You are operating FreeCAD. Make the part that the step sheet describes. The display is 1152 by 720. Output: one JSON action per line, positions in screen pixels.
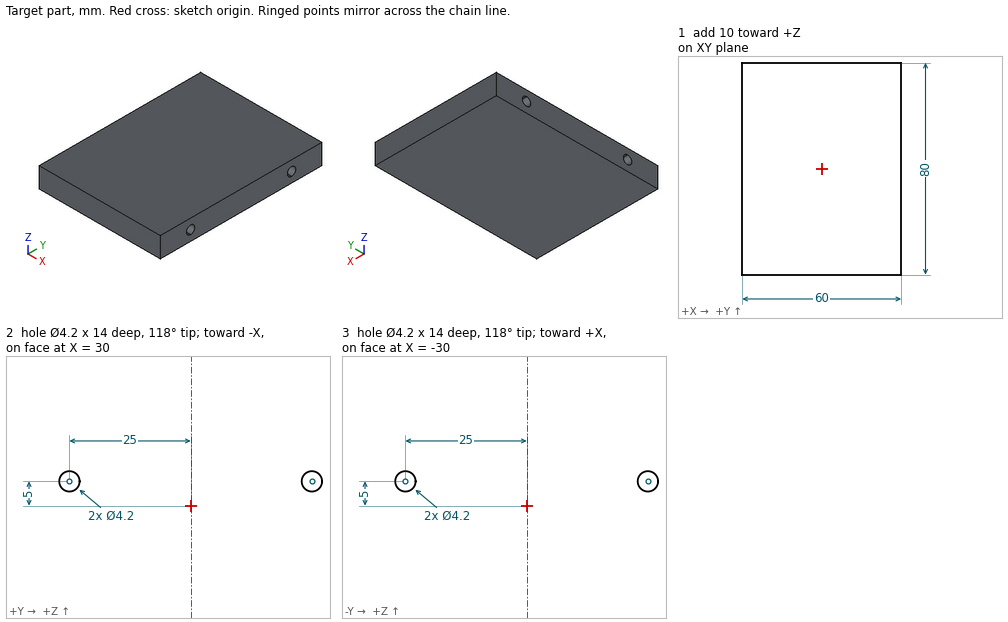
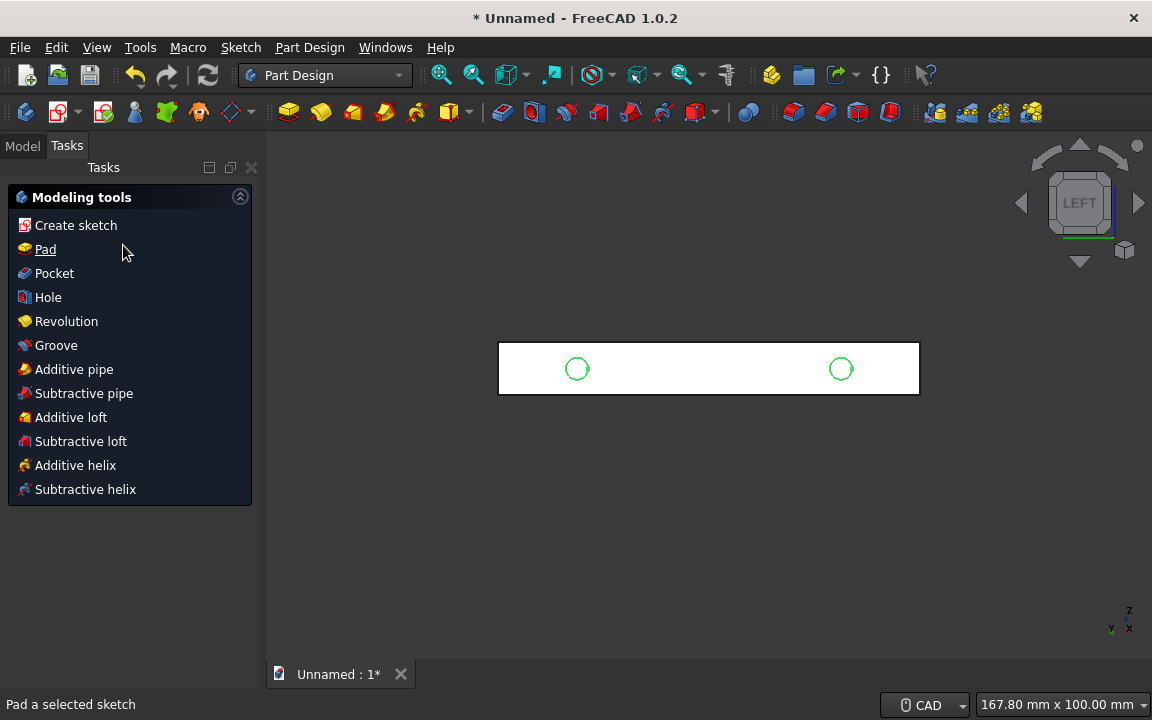
{"action": "left_click", "coordinate": [536, 112]}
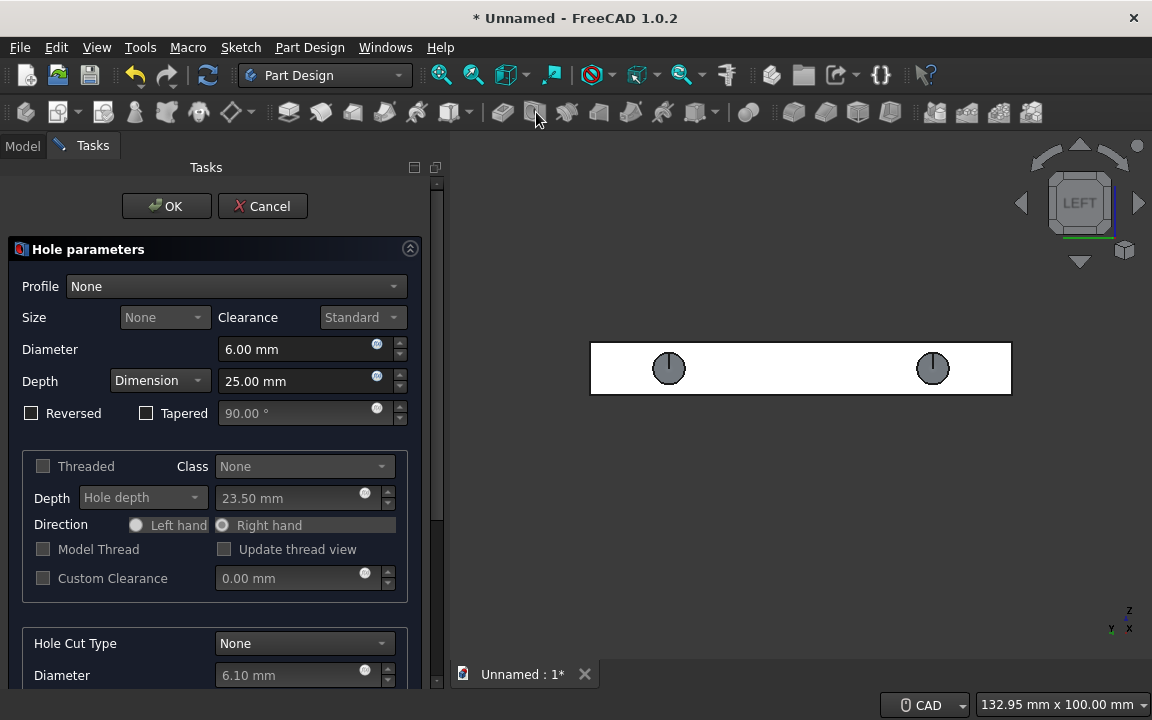
{"action": "triple_click", "coordinate": [305, 349]}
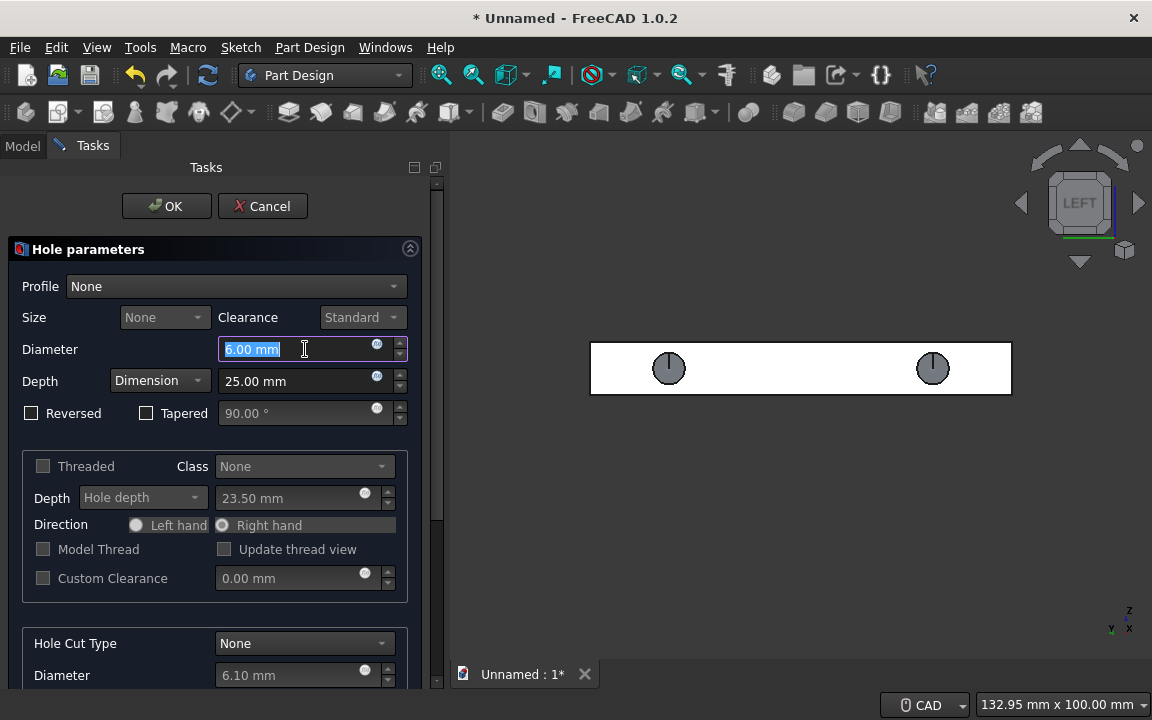
{"action": "type", "text": "4.2"}
{"action": "key", "text": "Tab"}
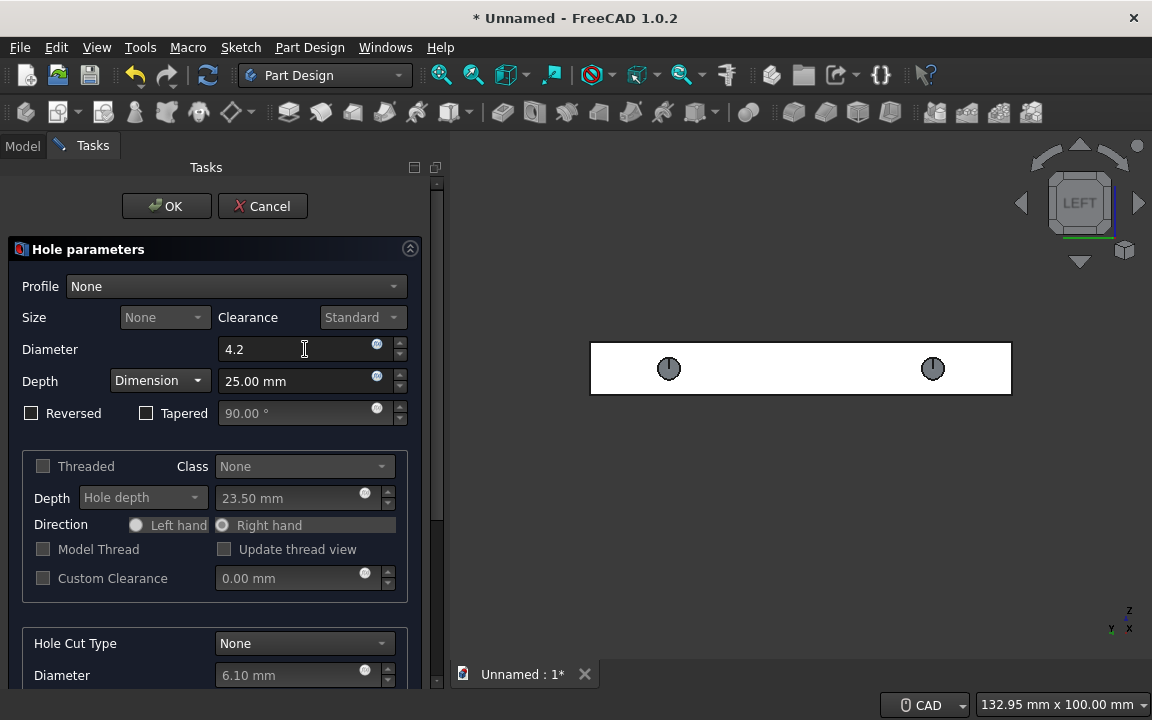
{"action": "triple_click", "coordinate": [305, 381]}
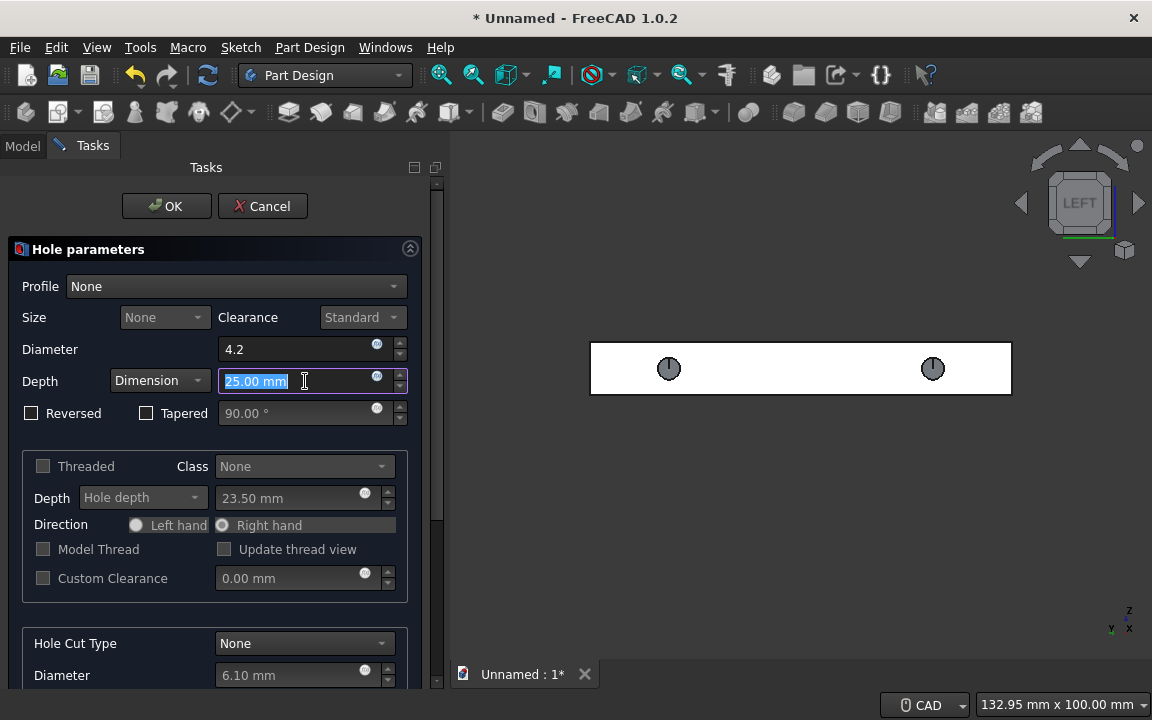
{"action": "type", "text": "14"}
{"action": "key", "text": "Tab"}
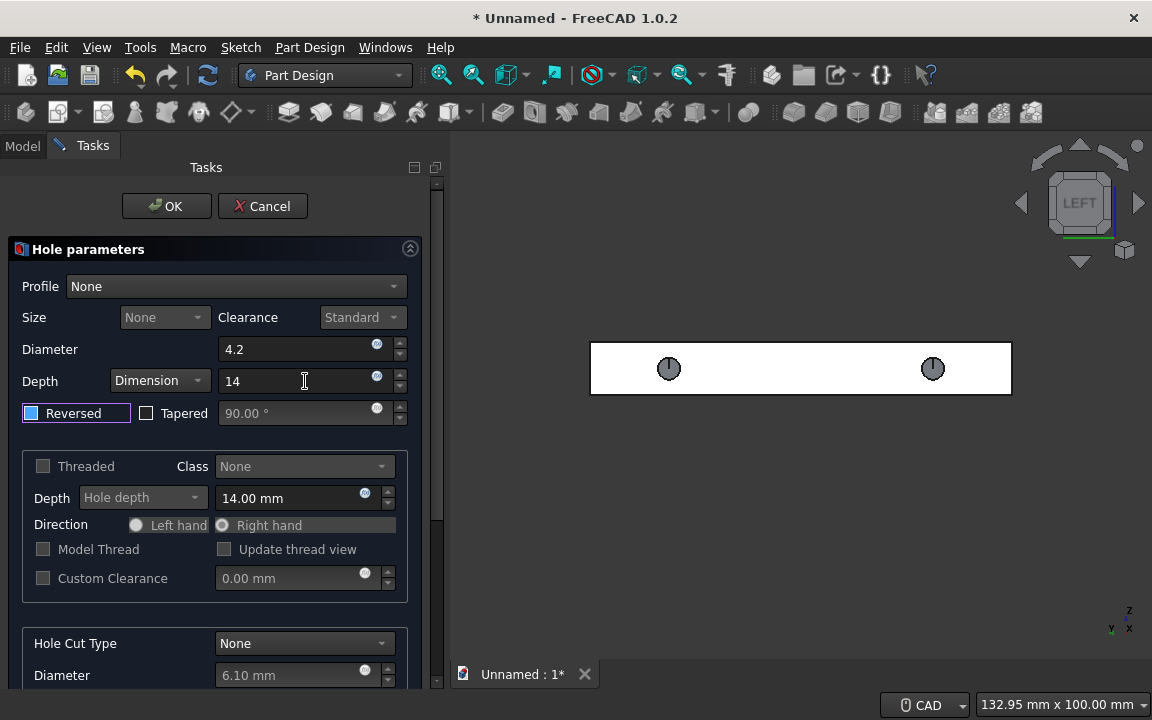
{"action": "left_click", "coordinate": [167, 206]}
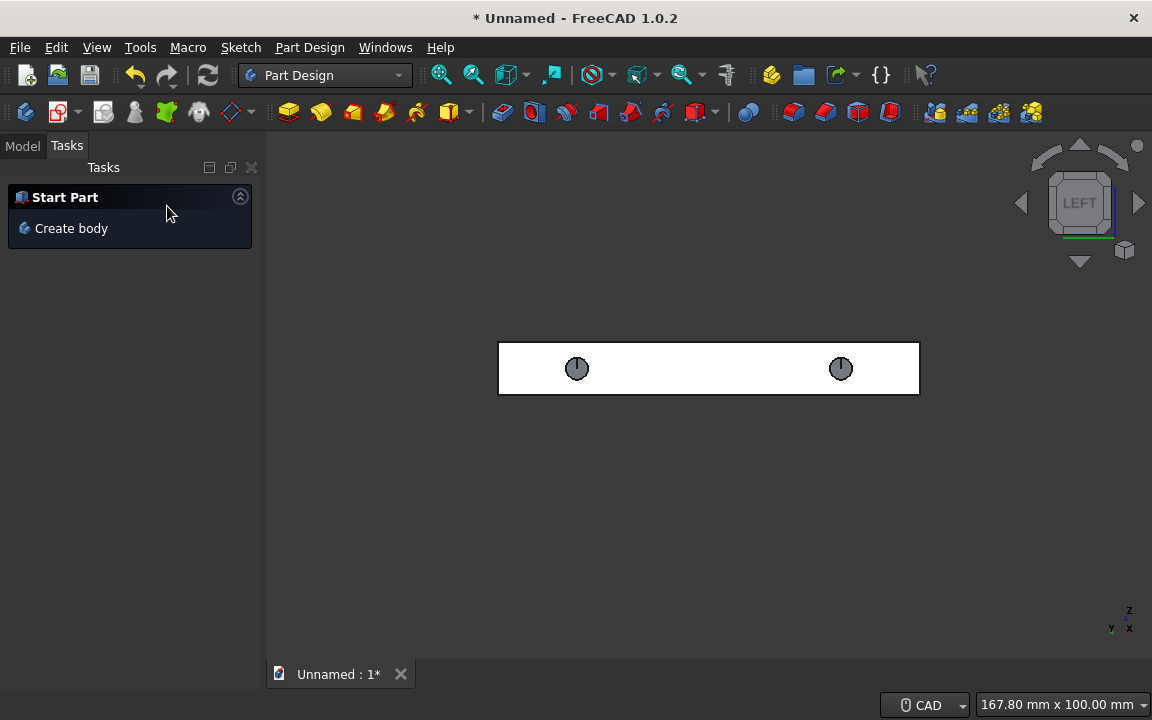
{"action": "key", "text": "0"}